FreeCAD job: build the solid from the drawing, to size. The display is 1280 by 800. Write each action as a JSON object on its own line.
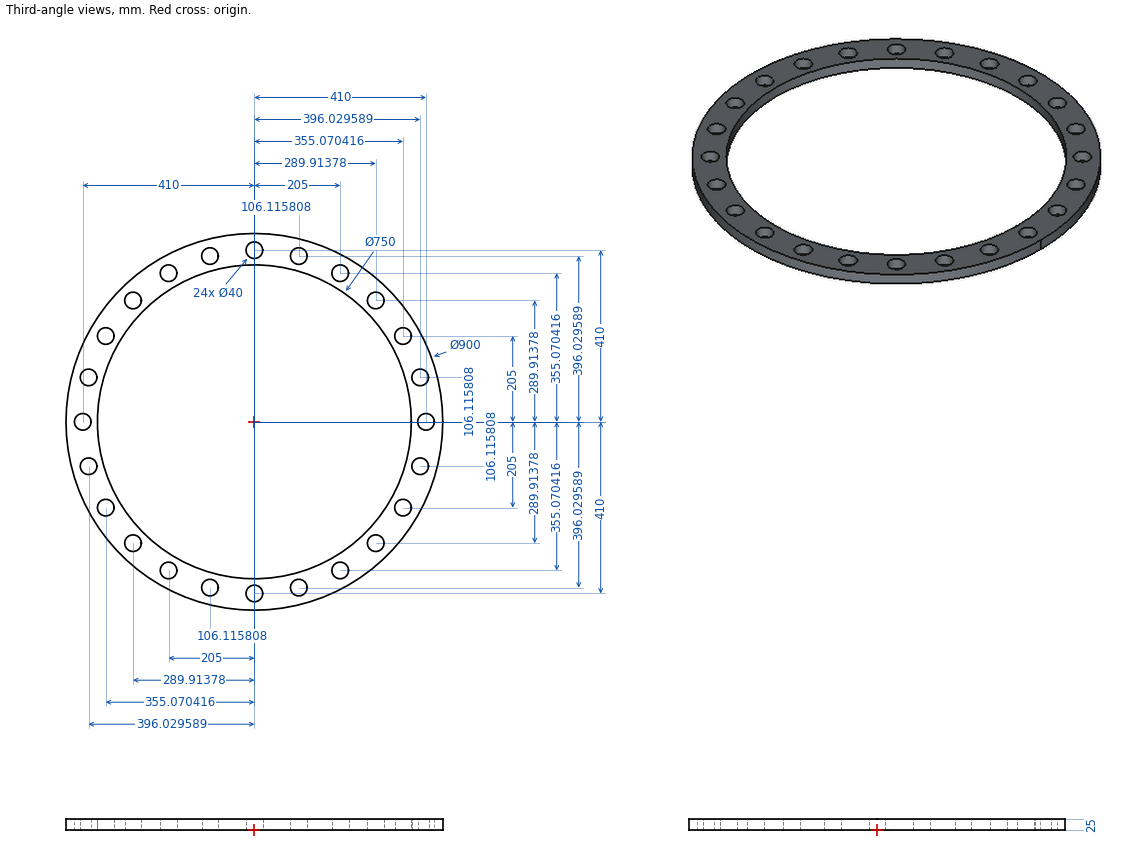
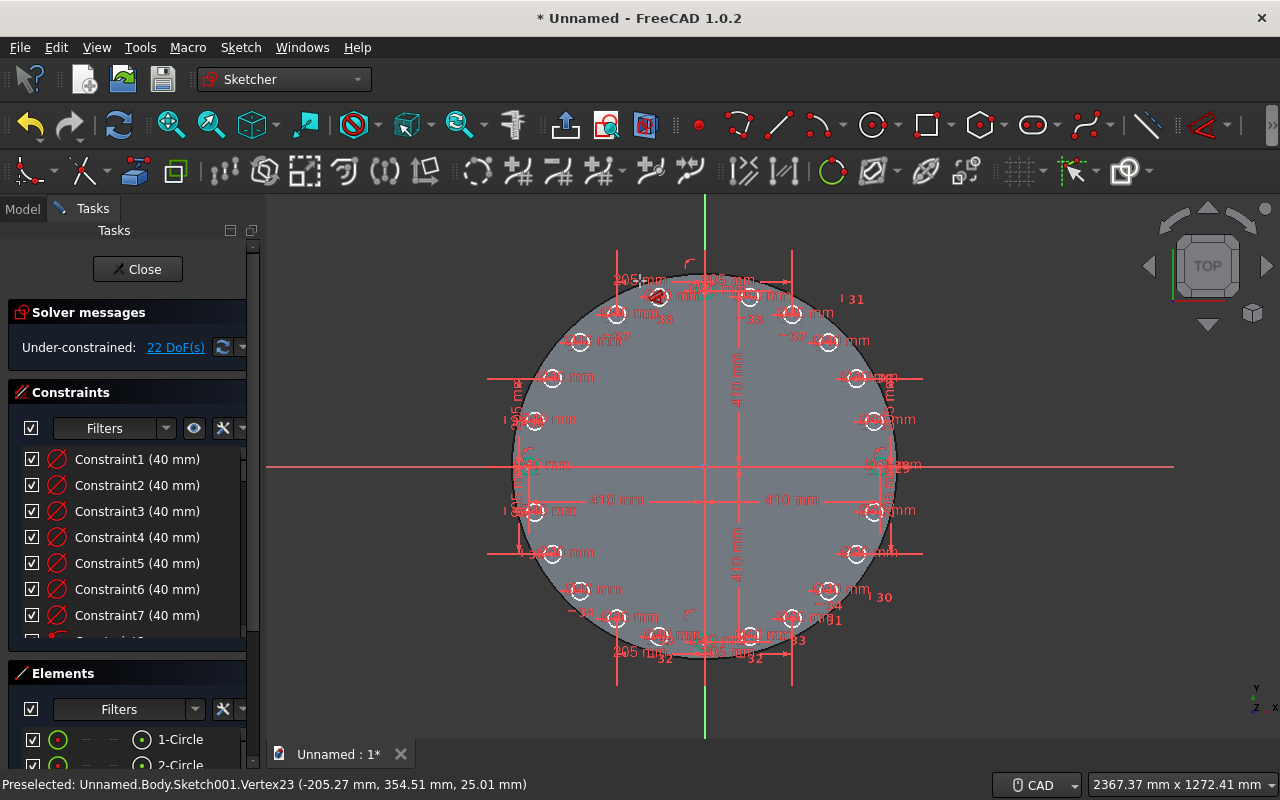
{"action": "left_click", "coordinate": [829, 343]}
{"action": "left_click", "coordinate": [723, 309]}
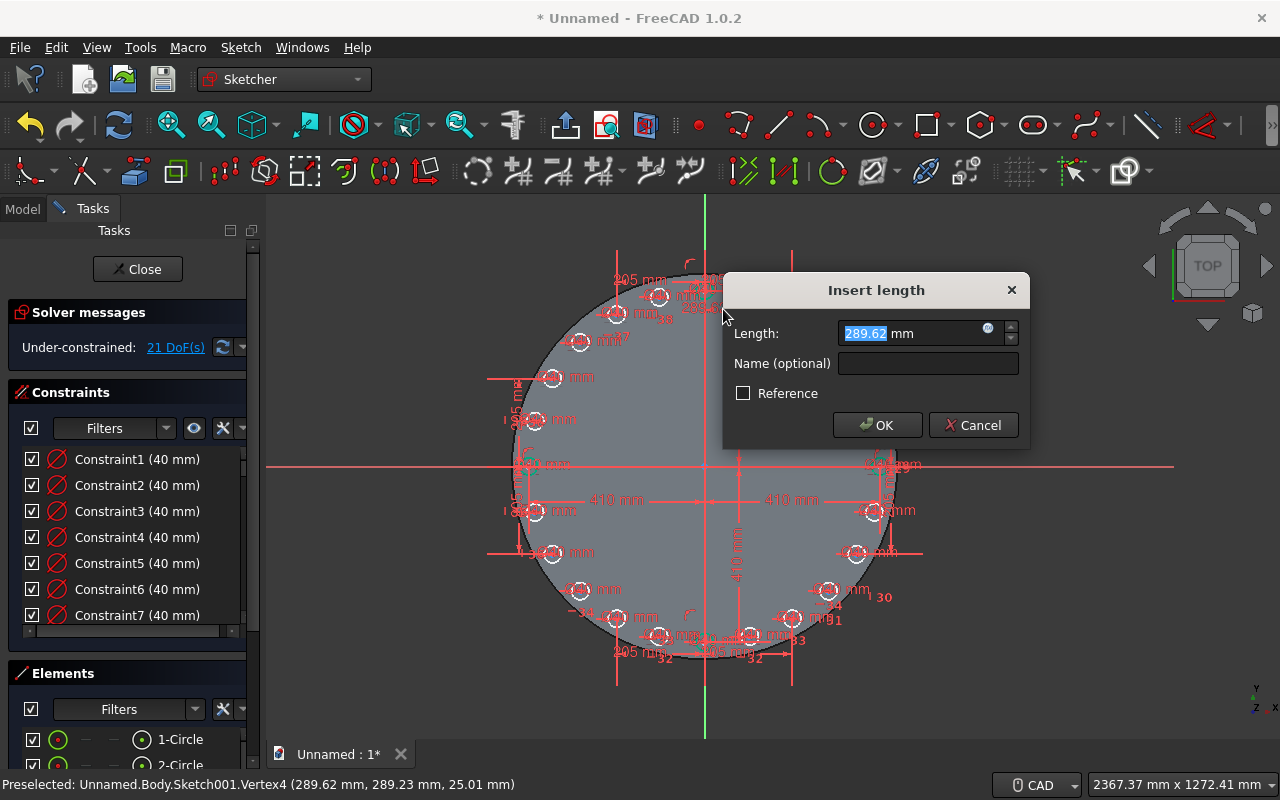
{"action": "type", "text": "289.91378"}
{"action": "key", "text": "Return"}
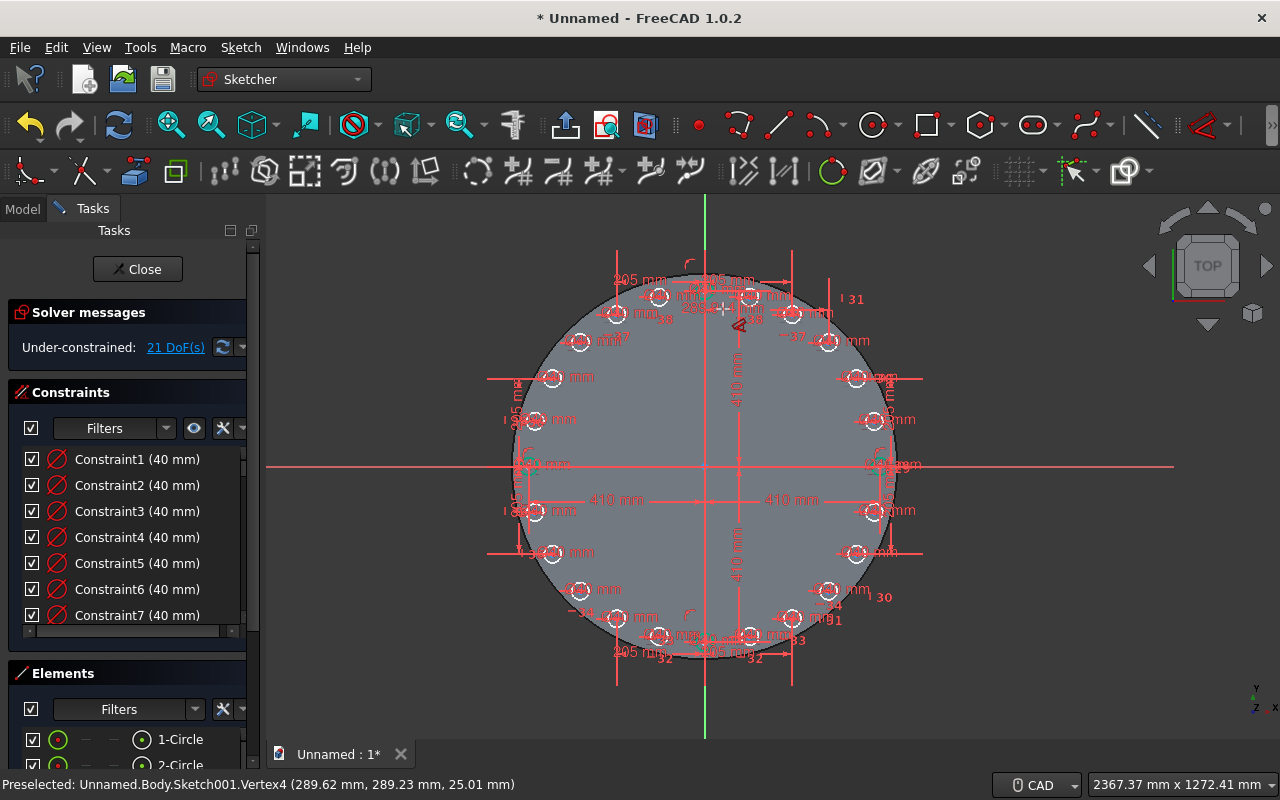
{"action": "left_click", "coordinate": [829, 343]}
{"action": "left_click", "coordinate": [863, 448]}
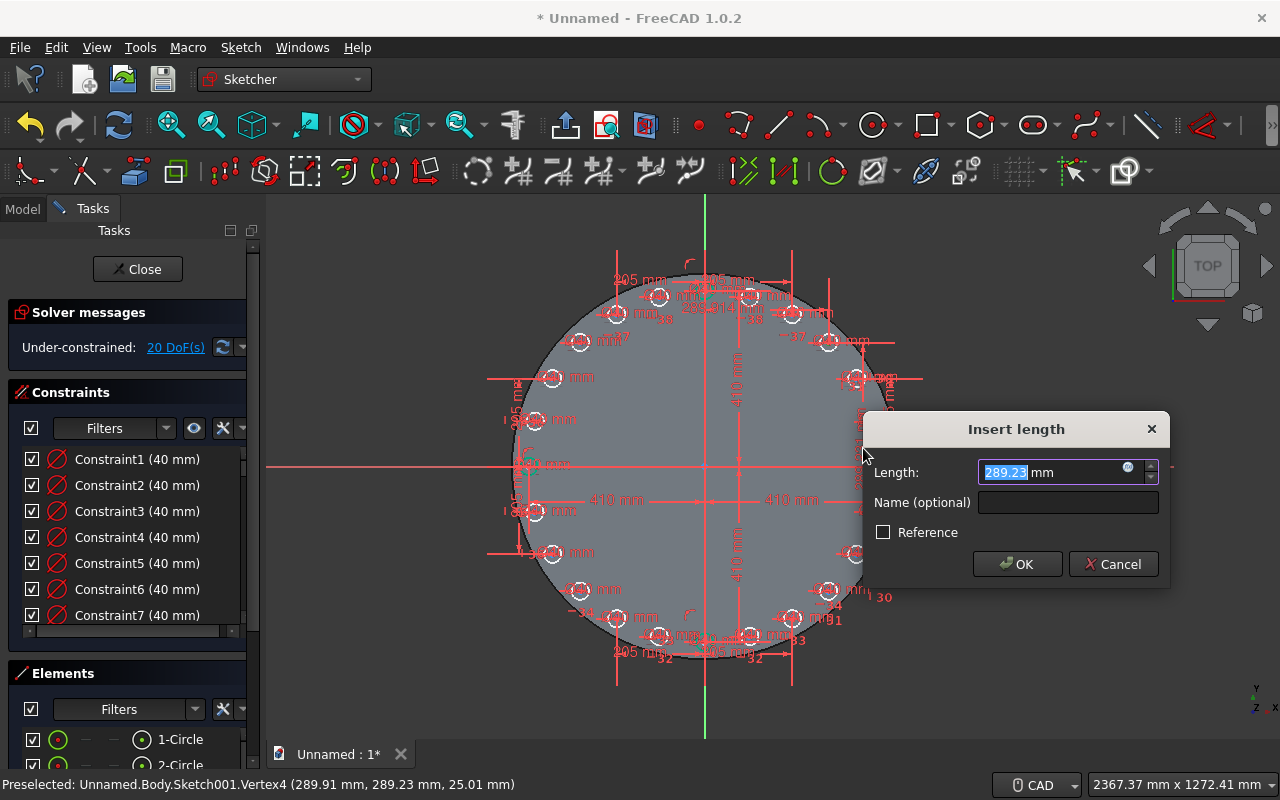
{"action": "type", "text": "289.91378"}
{"action": "key", "text": "Return"}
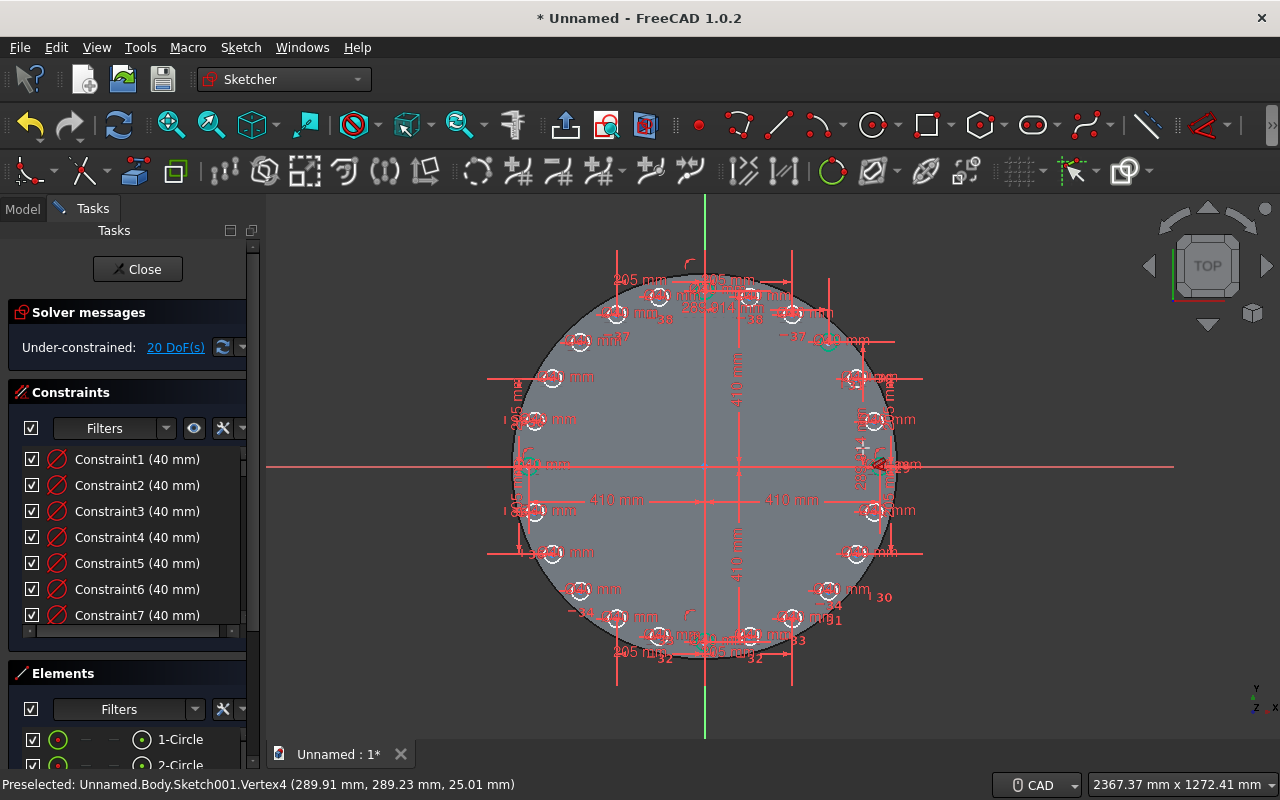
{"action": "left_click", "coordinate": [829, 591]}
{"action": "left_click", "coordinate": [671, 529]}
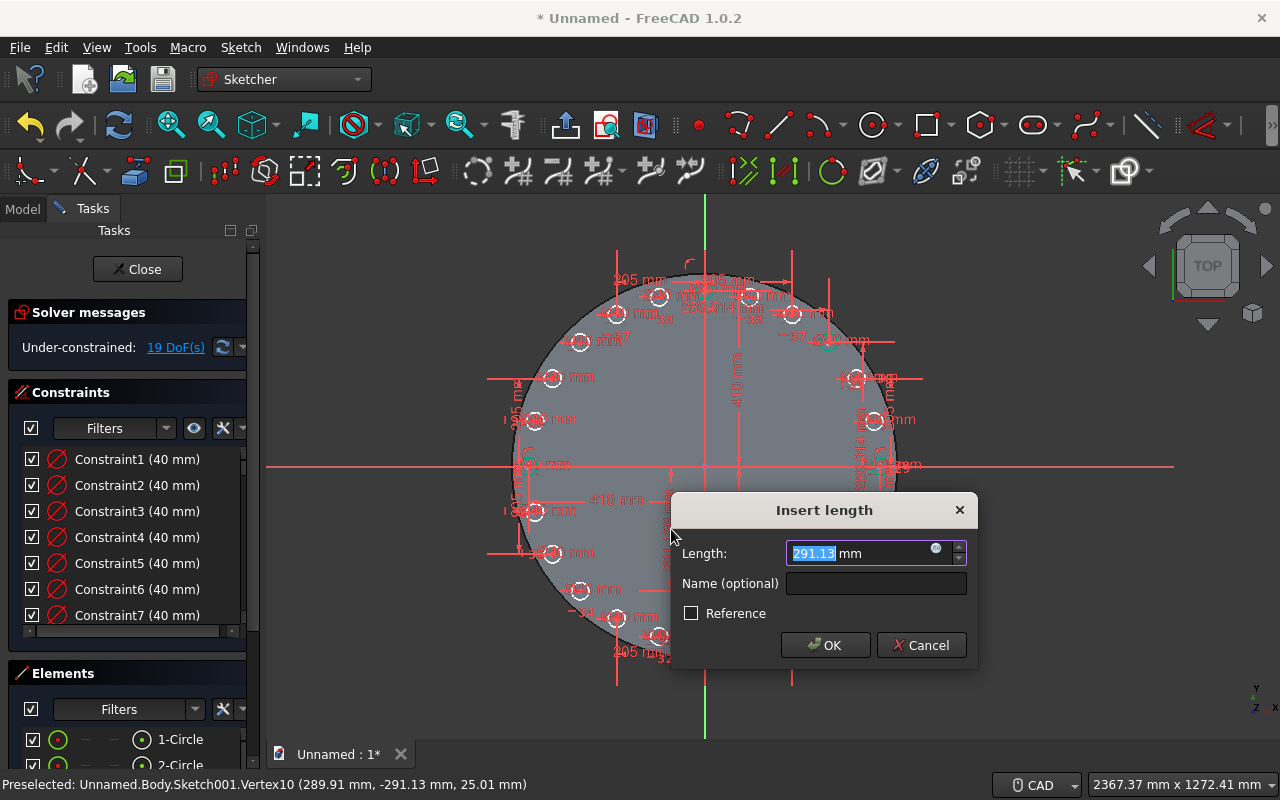
{"action": "type", "text": "289.91378"}
{"action": "key", "text": "Return"}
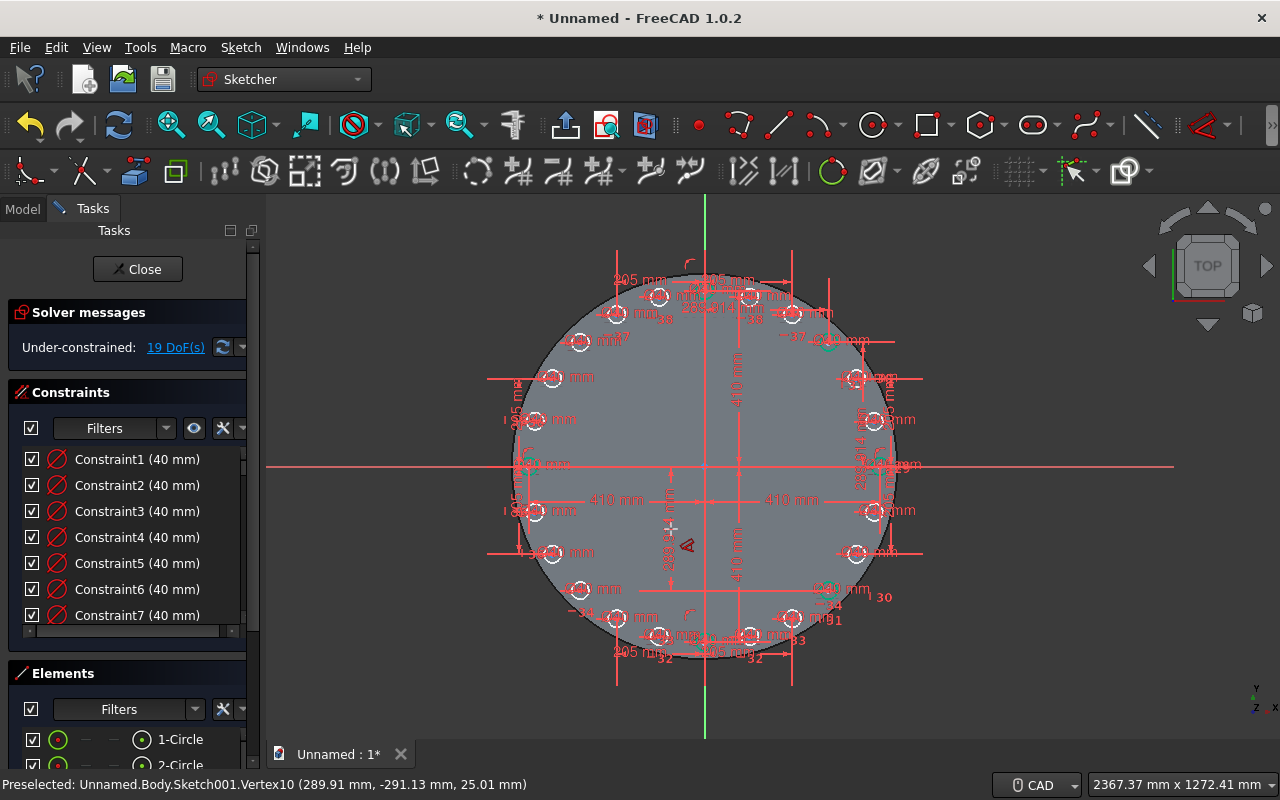
{"action": "left_click", "coordinate": [580, 591]}
{"action": "left_click", "coordinate": [686, 625]}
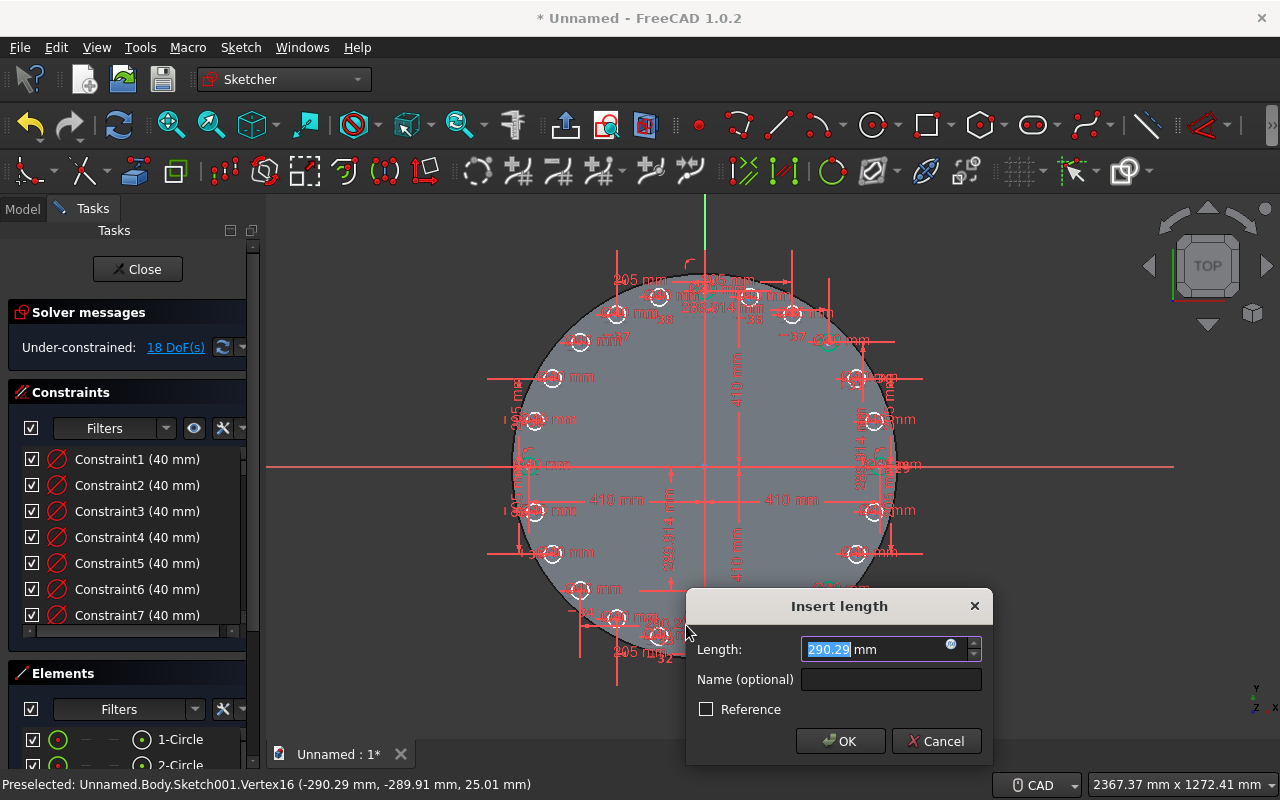
{"action": "type", "text": "289.91378"}
{"action": "key", "text": "Return"}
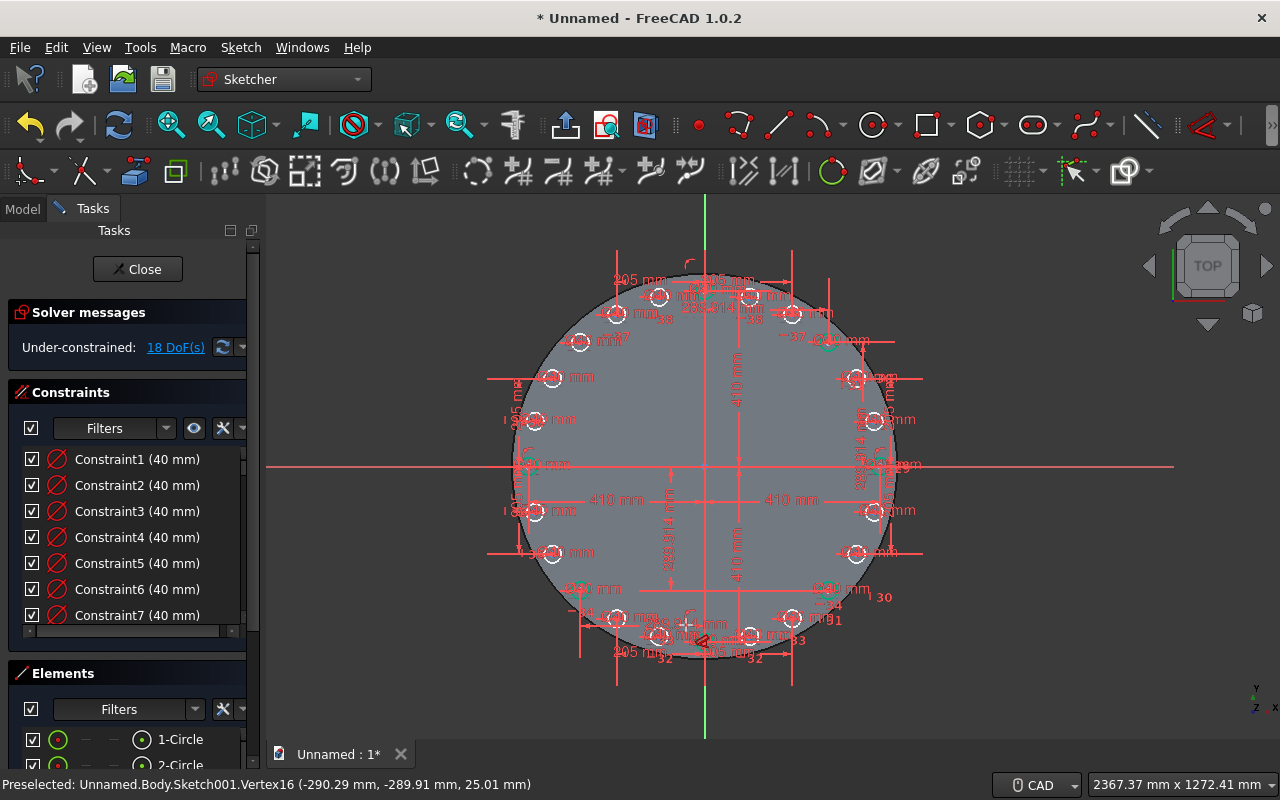
{"action": "left_click", "coordinate": [580, 343]}
{"action": "left_click", "coordinate": [599, 525]}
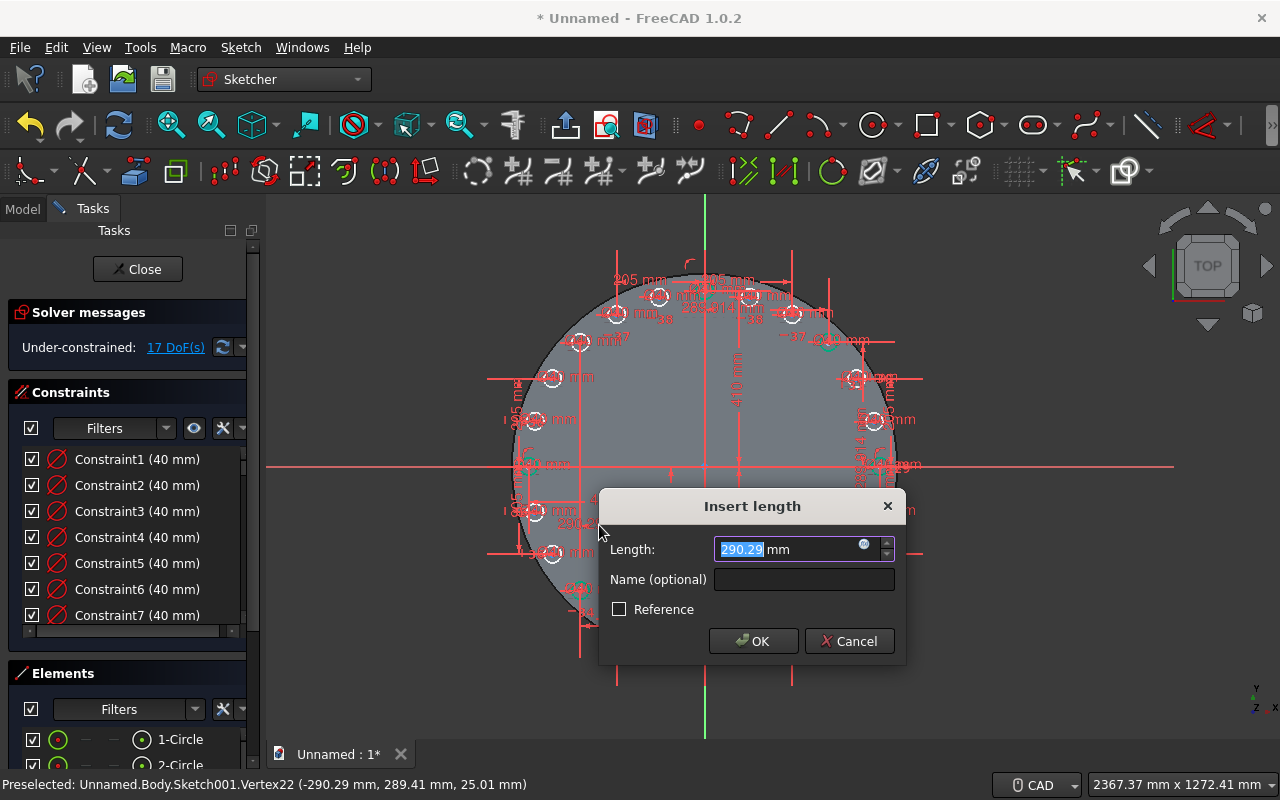
{"action": "type", "text": "289.91378"}
{"action": "key", "text": "Return"}